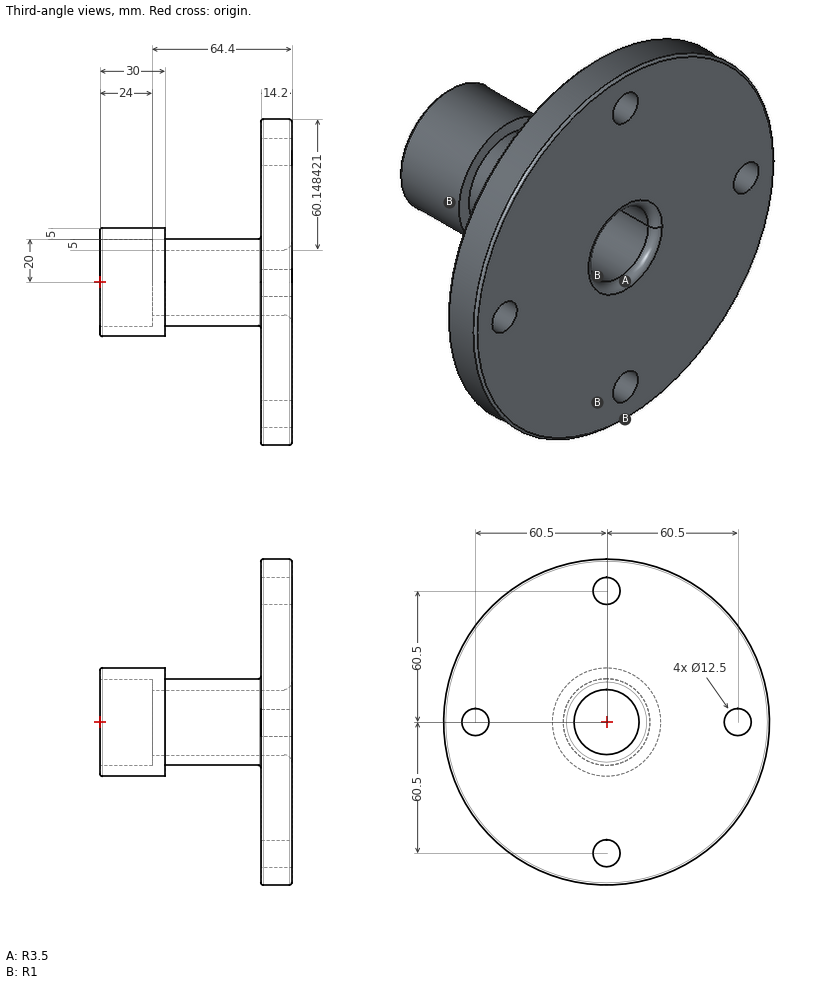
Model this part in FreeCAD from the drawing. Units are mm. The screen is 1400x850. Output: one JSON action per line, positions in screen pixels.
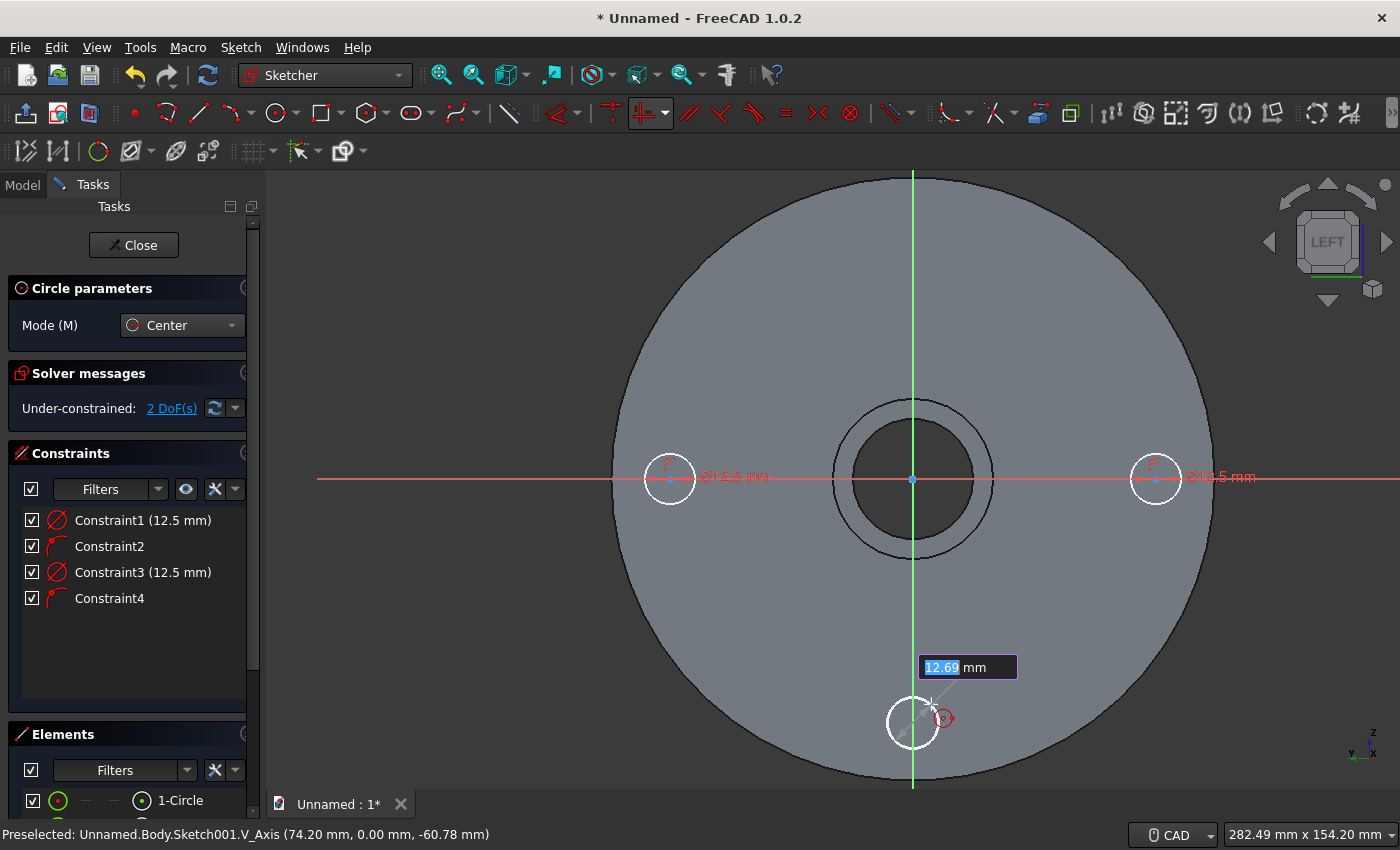
{"action": "type", "text": "12.5"}
{"action": "key", "text": "Return"}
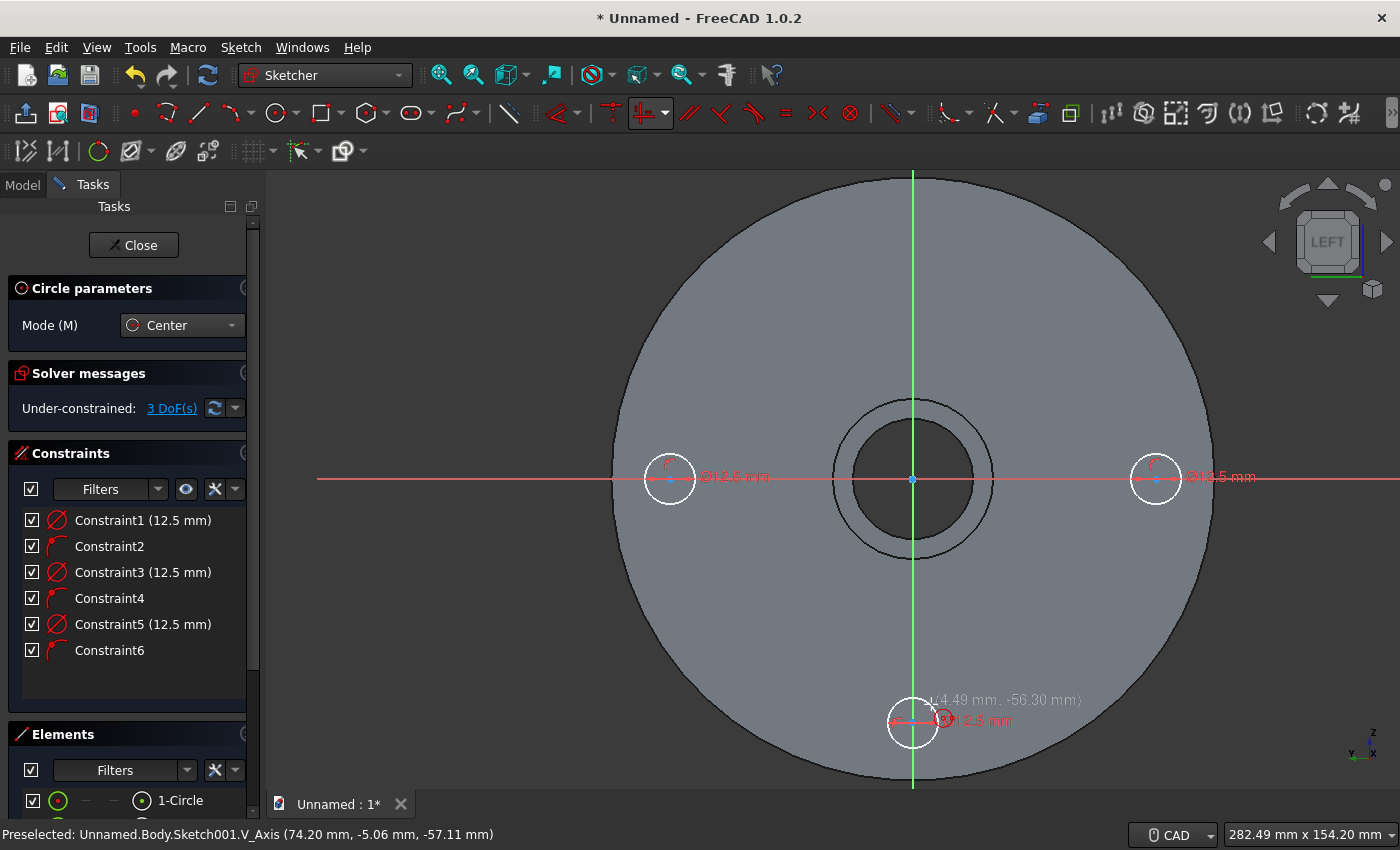
{"action": "left_click", "coordinate": [913, 236]}
{"action": "mouse_move", "coordinate": [931, 218]}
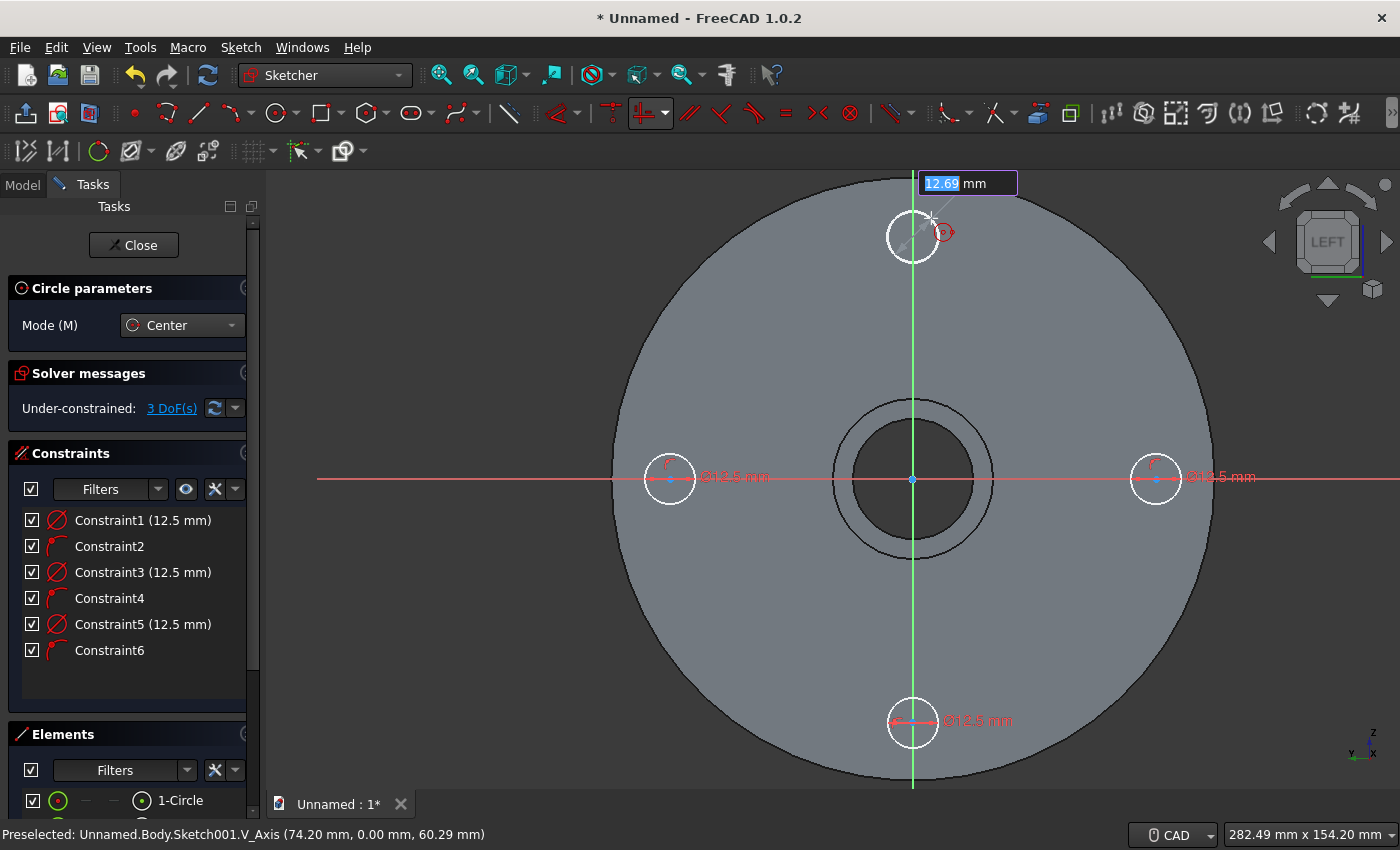
{"action": "type", "text": "12.5"}
{"action": "key", "text": "Return"}
{"action": "key", "text": "Escape"}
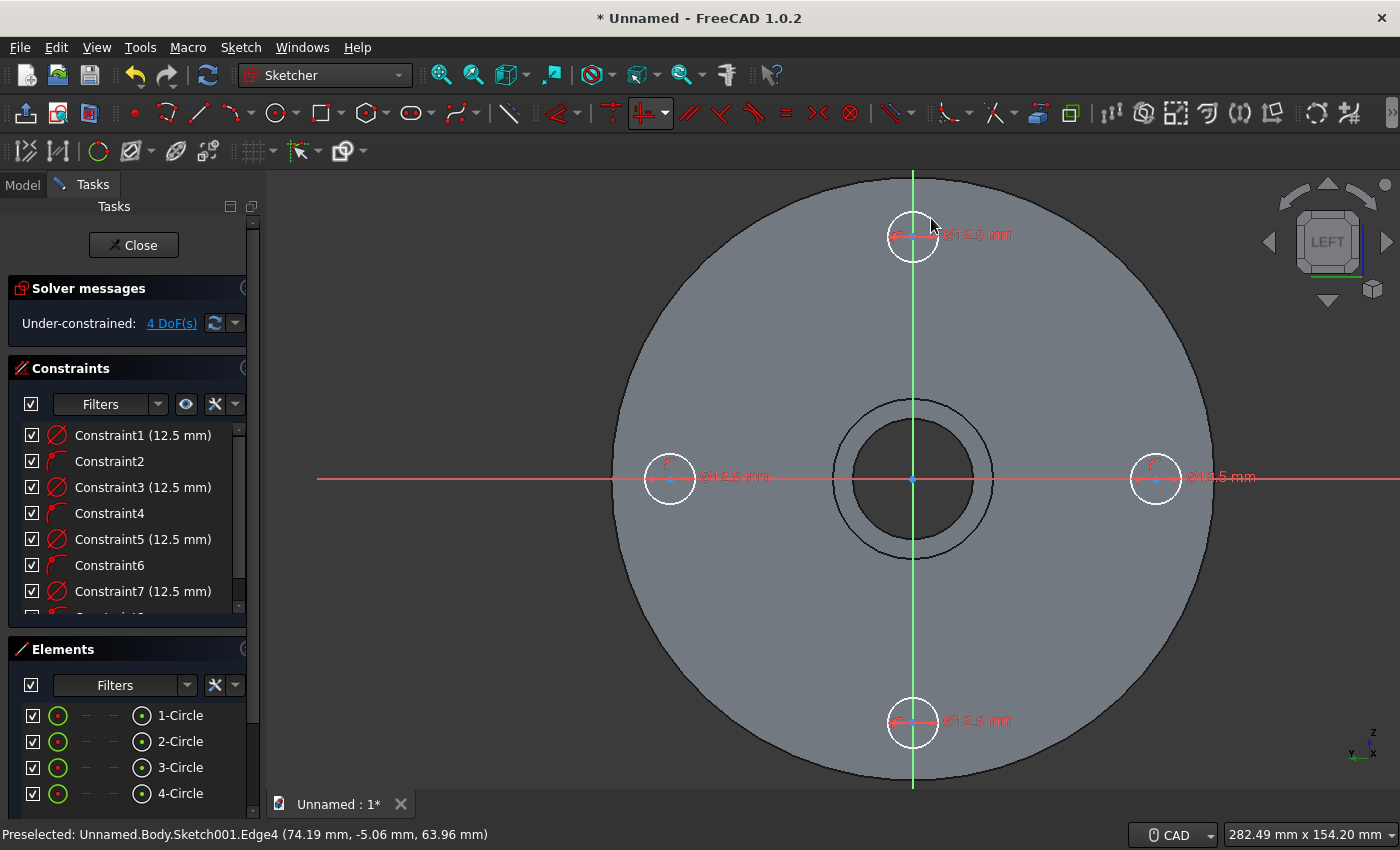
{"action": "left_click", "coordinate": [556, 114]}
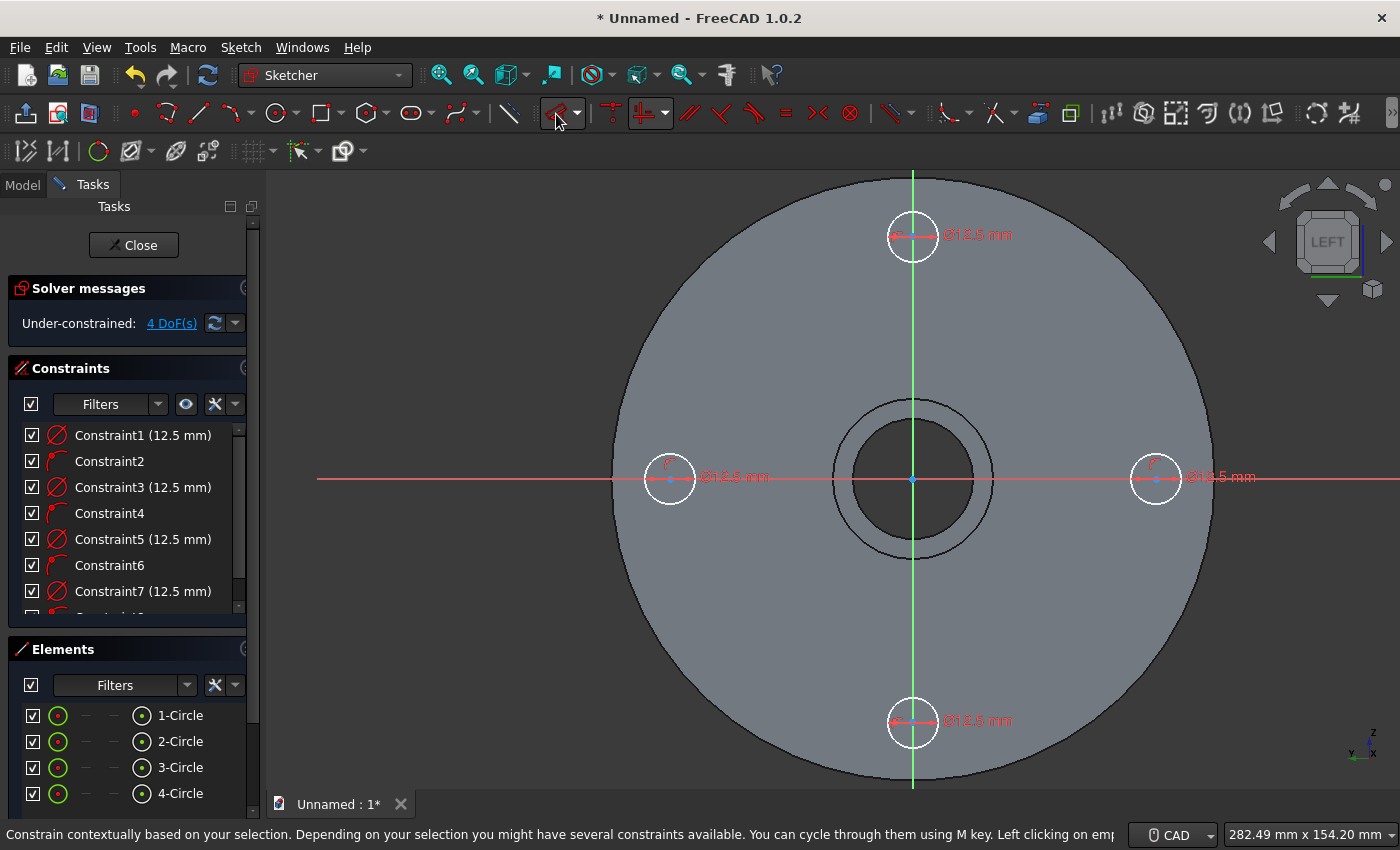
{"action": "left_click", "coordinate": [670, 479]}
{"action": "left_click", "coordinate": [791, 513]}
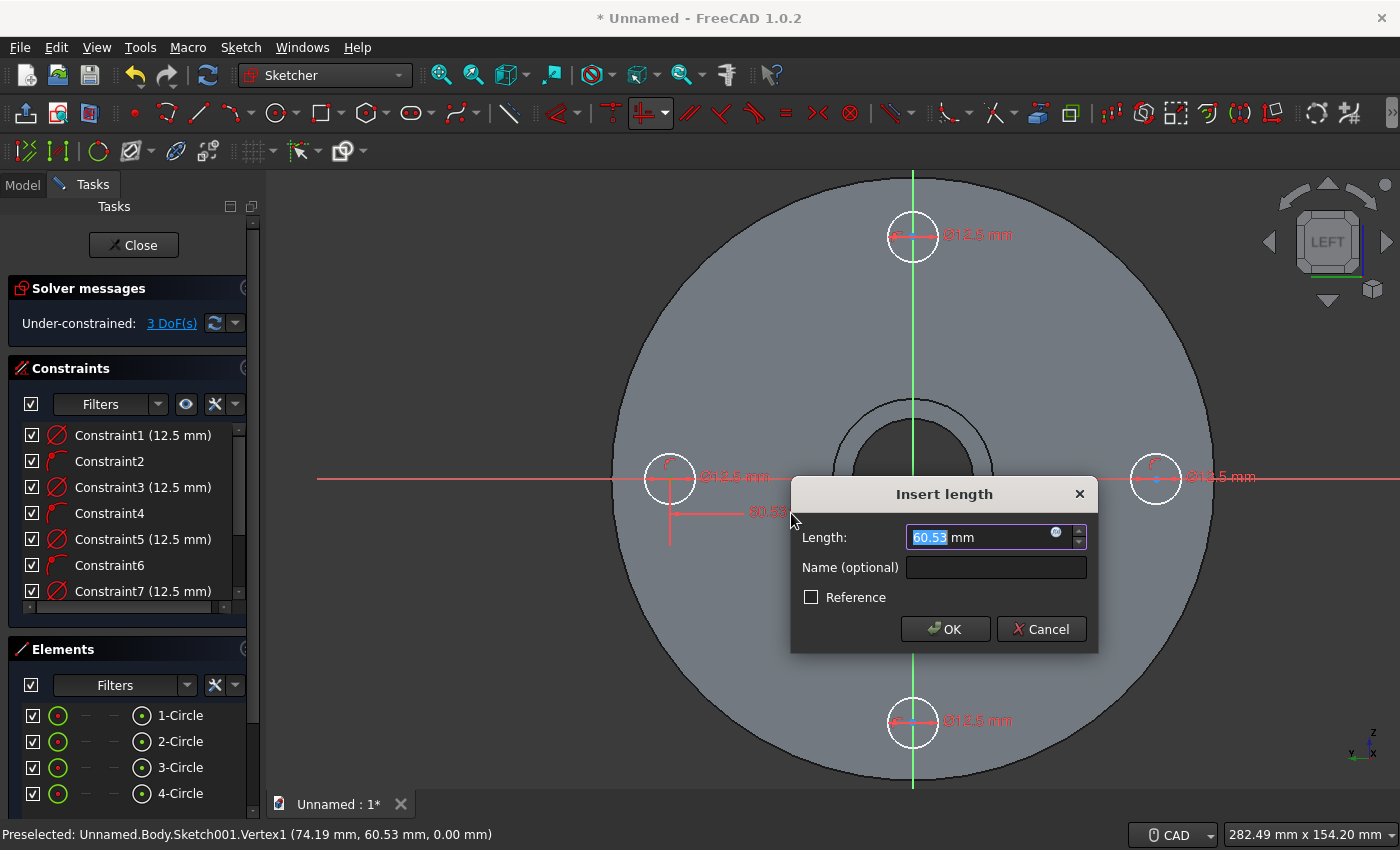
{"action": "type", "text": "60.5"}
{"action": "key", "text": "Return"}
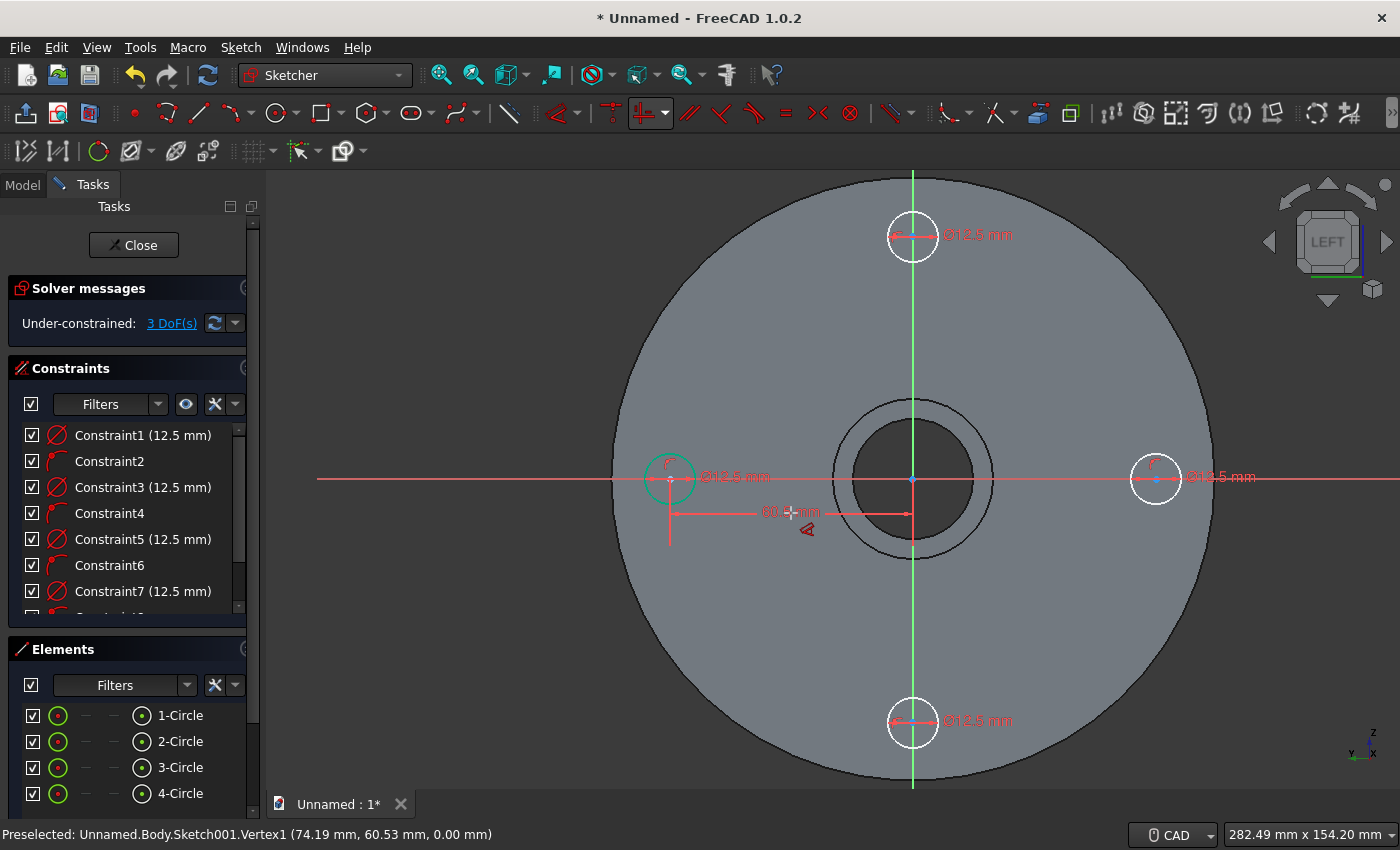
{"action": "left_click", "coordinate": [1156, 479]}
{"action": "left_click", "coordinate": [1034, 513]}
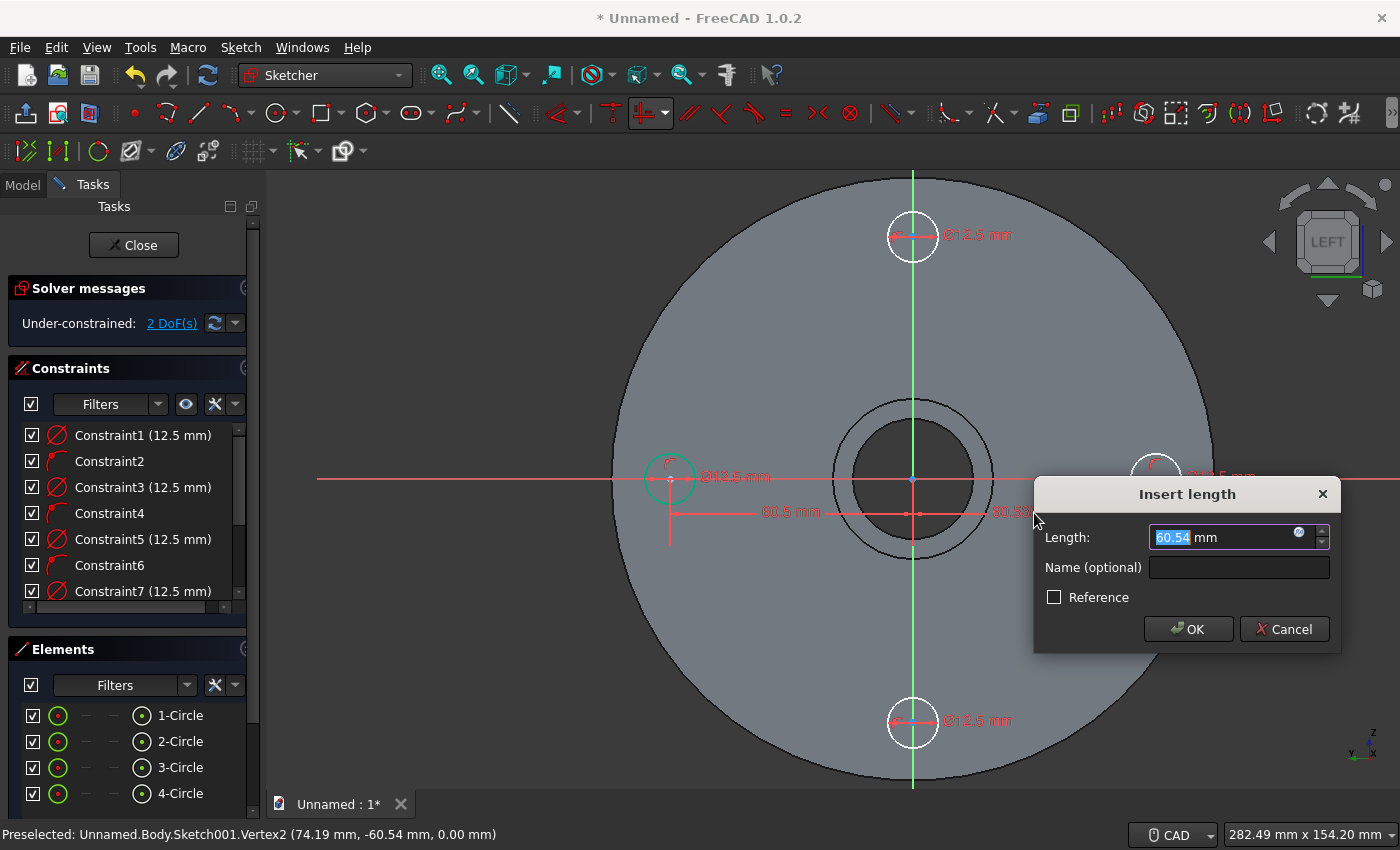
{"action": "type", "text": "60.5"}
{"action": "key", "text": "Return"}